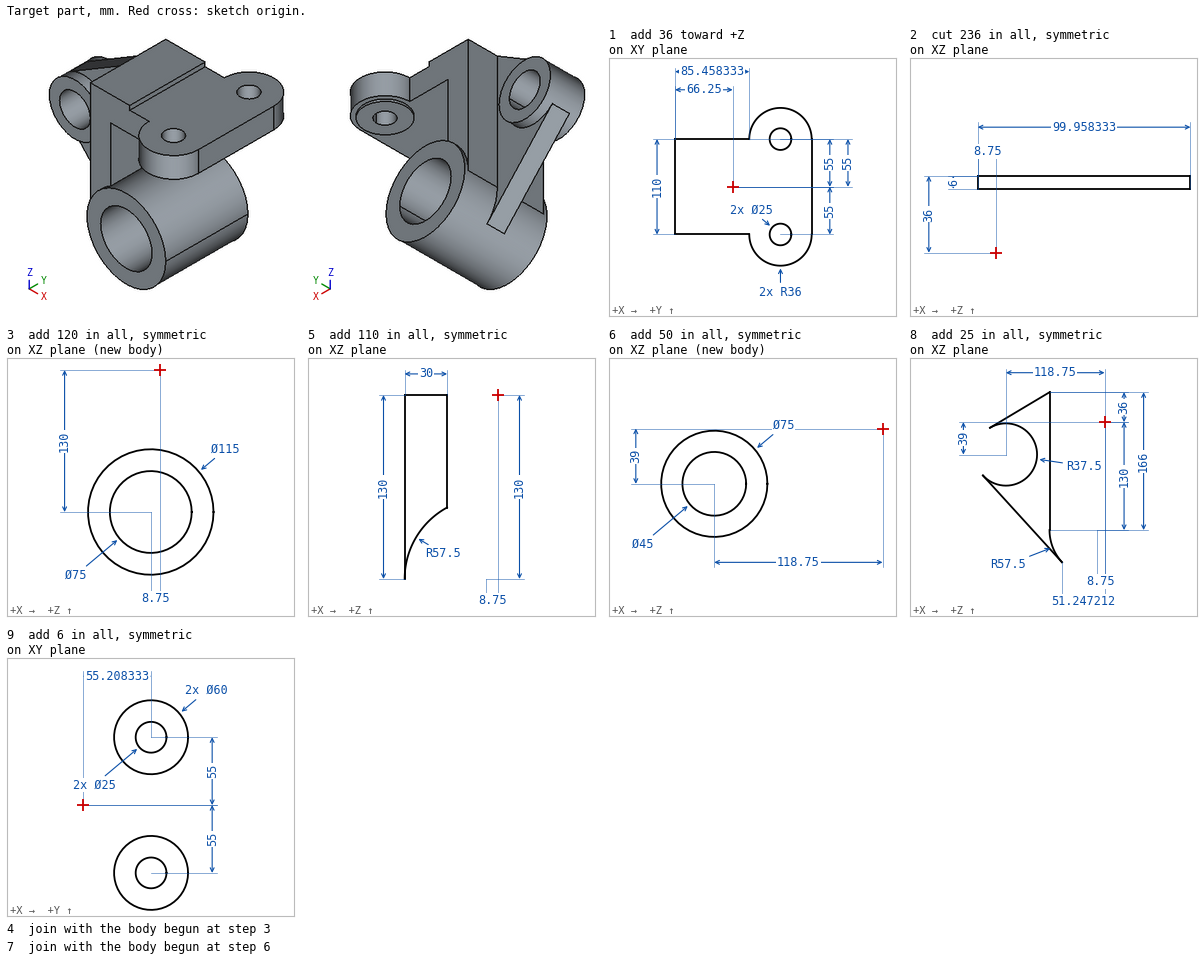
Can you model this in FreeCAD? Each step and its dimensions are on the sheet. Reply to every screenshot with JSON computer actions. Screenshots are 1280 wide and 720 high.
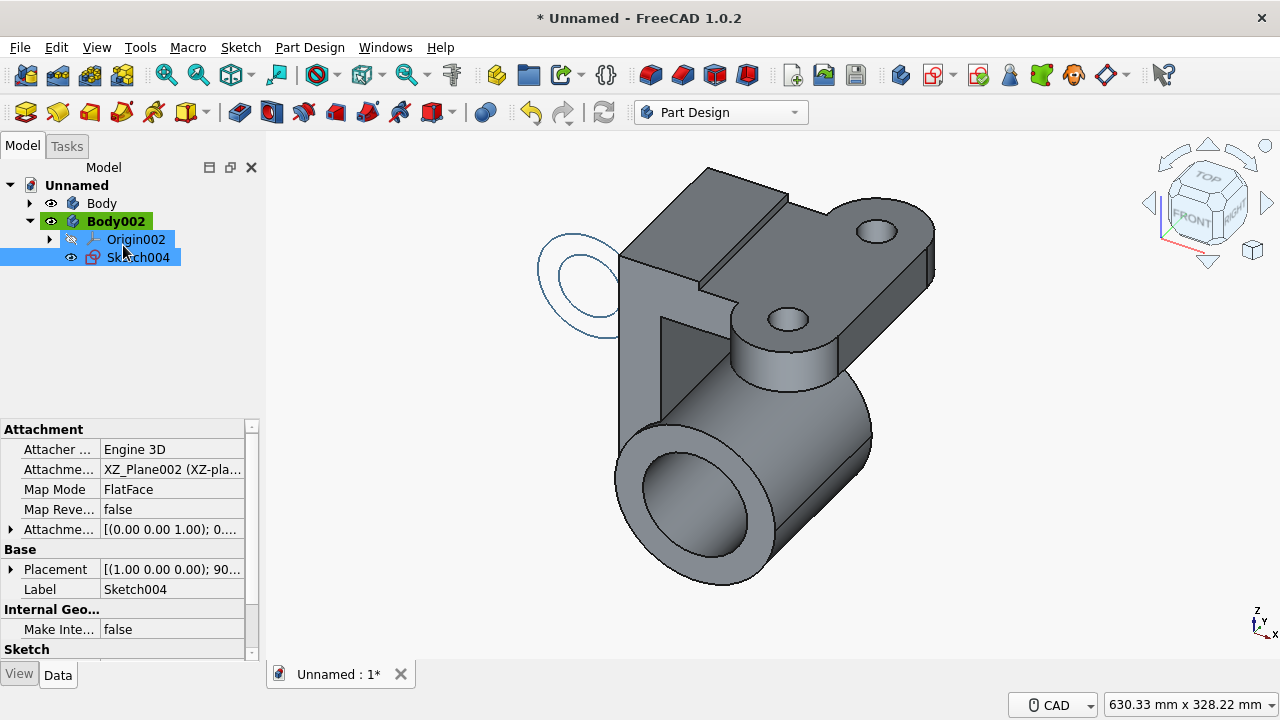
{"action": "left_click", "coordinate": [26, 112]}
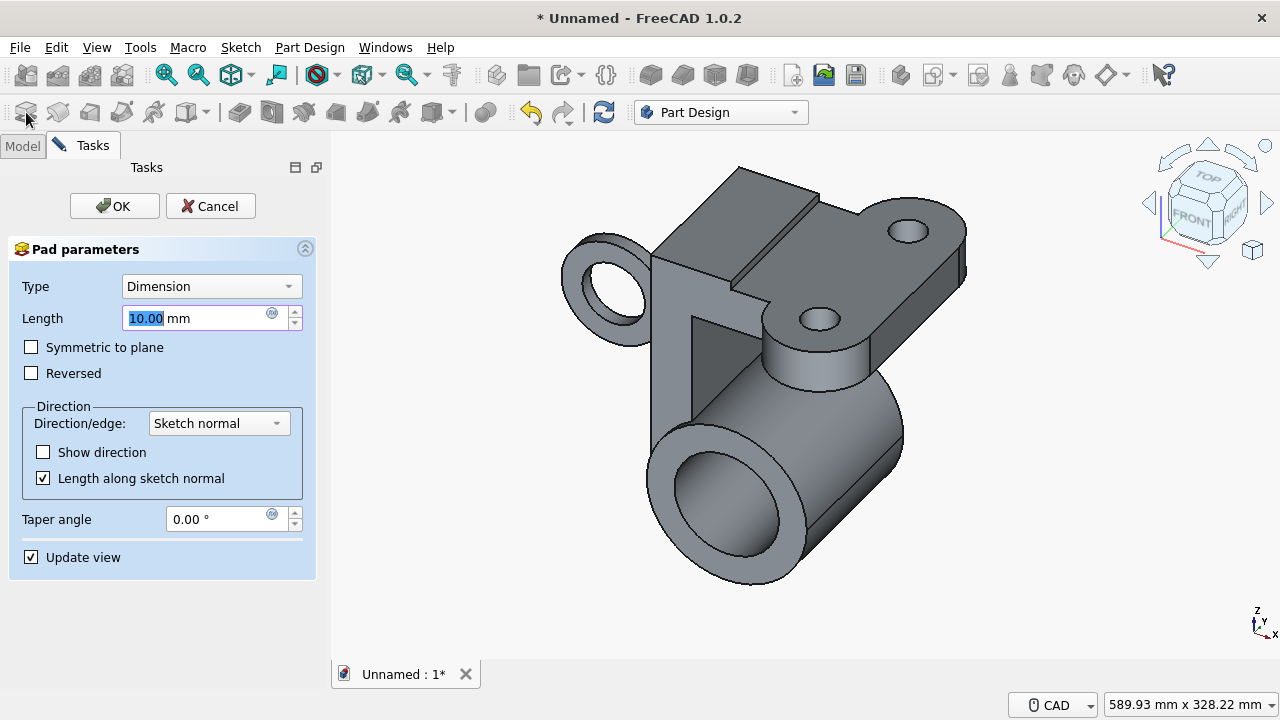
{"action": "type", "text": "50"}
{"action": "key", "text": "Tab"}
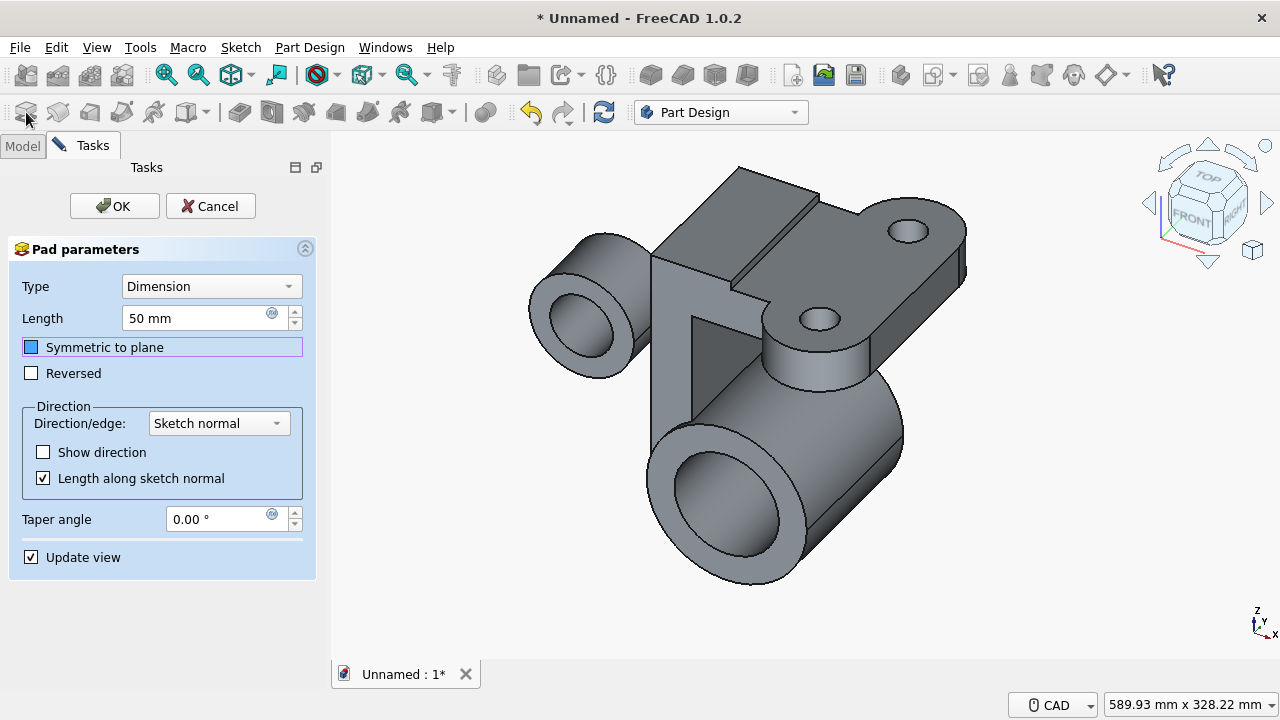
{"action": "left_click", "coordinate": [30, 347]}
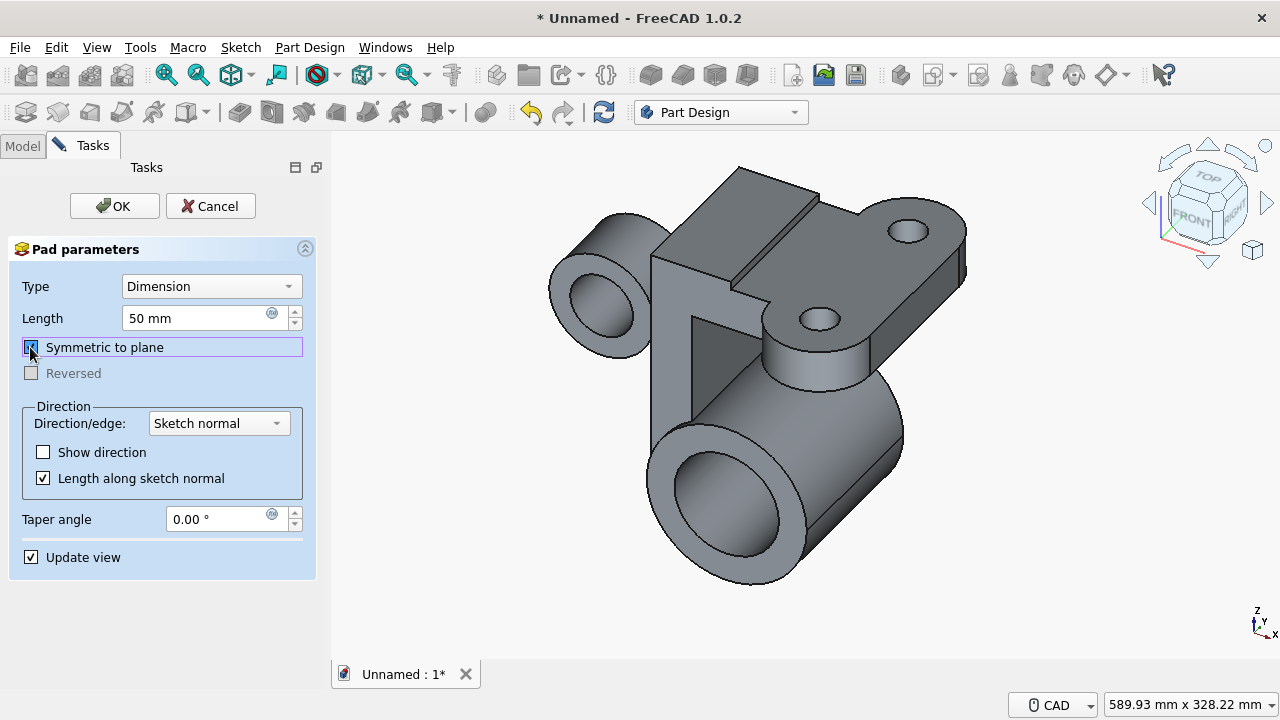
{"action": "left_click", "coordinate": [115, 206]}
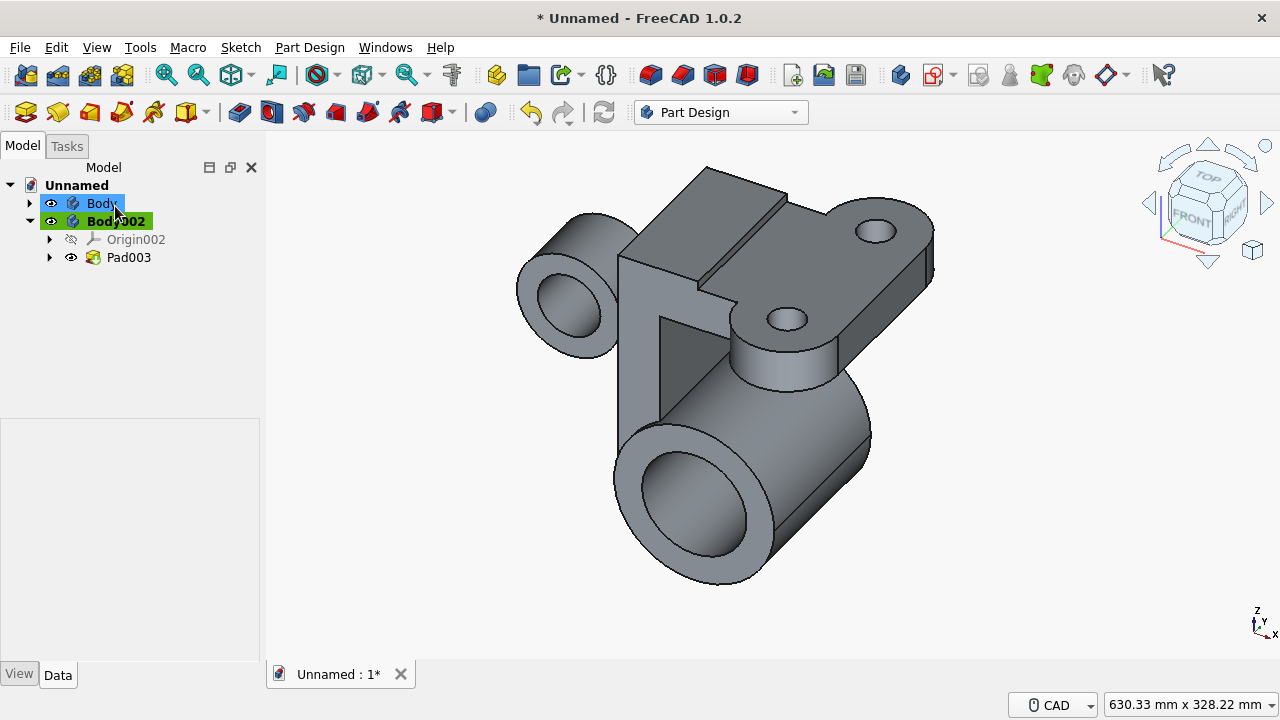
{"action": "key", "text": "v f"}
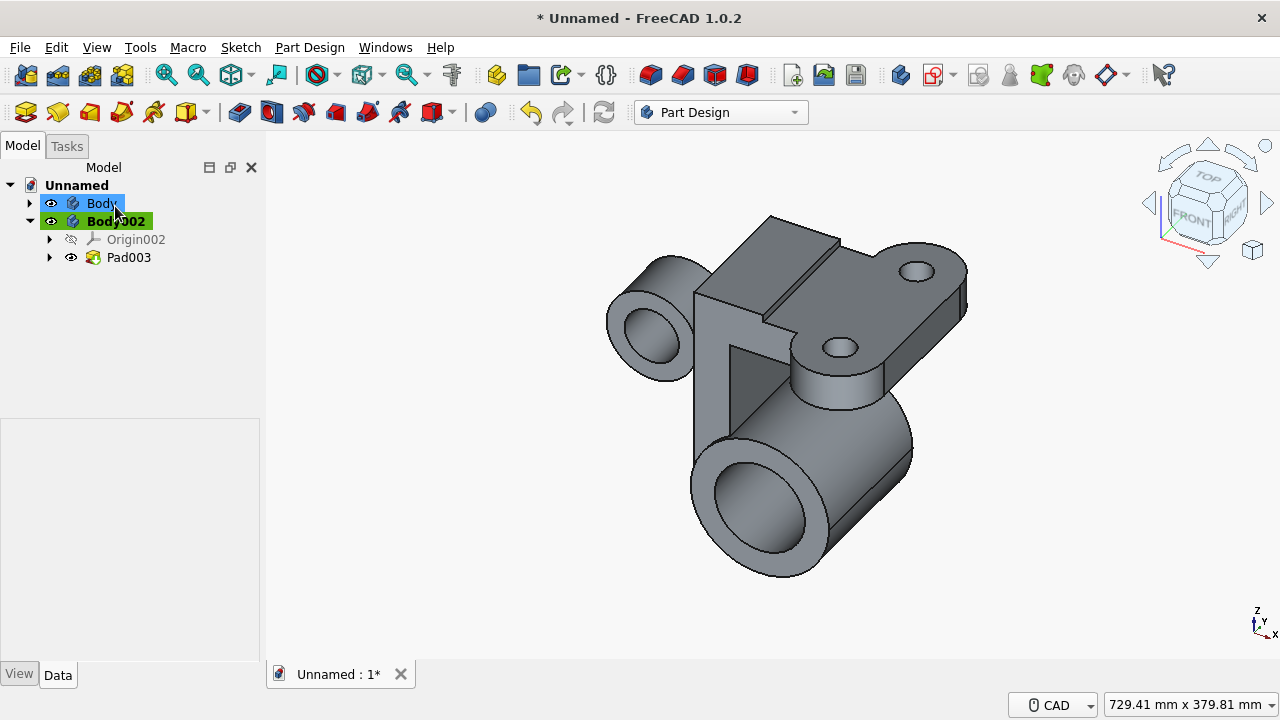
{"action": "double_click", "coordinate": [96, 203]}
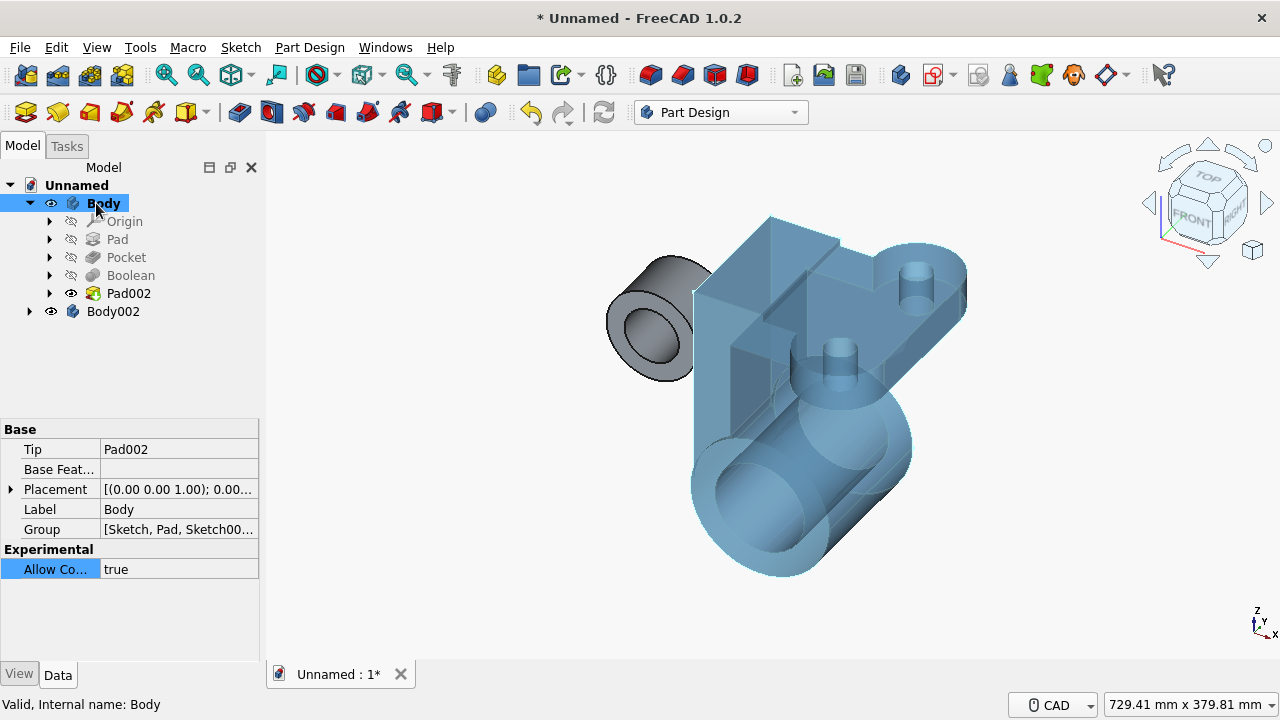
{"action": "left_click", "coordinate": [96, 311]}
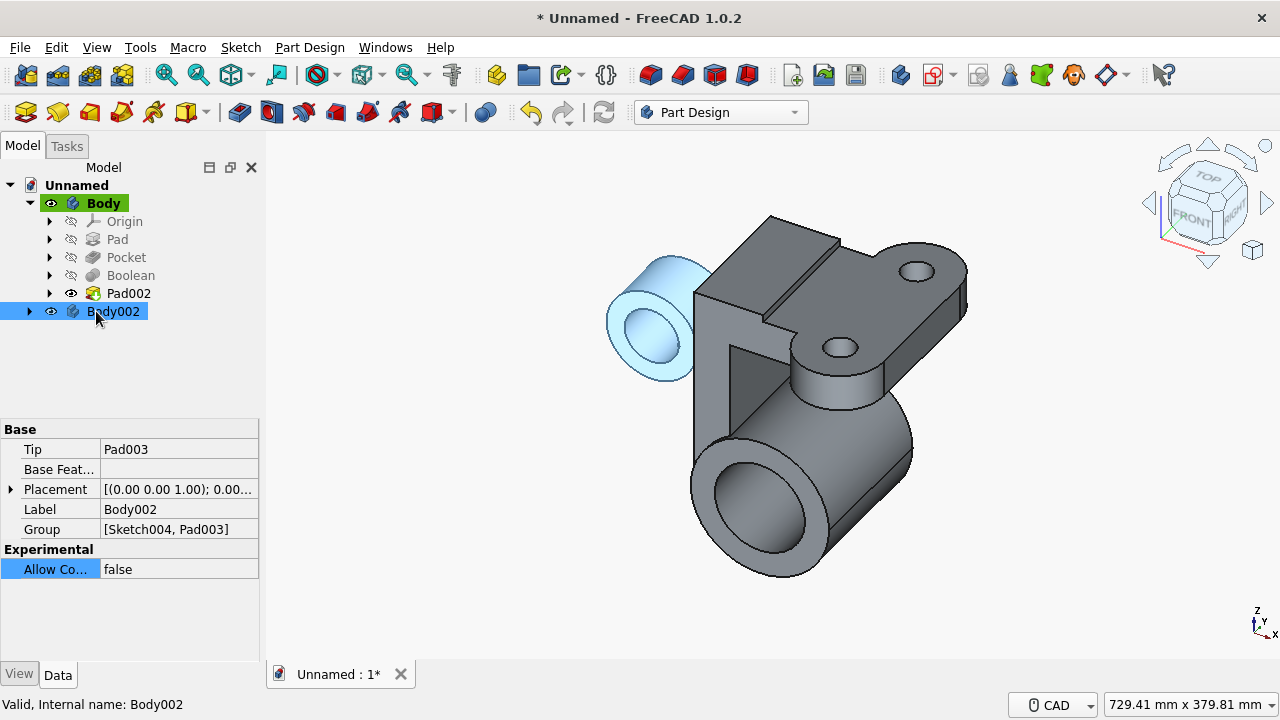
{"action": "left_click", "coordinate": [486, 112]}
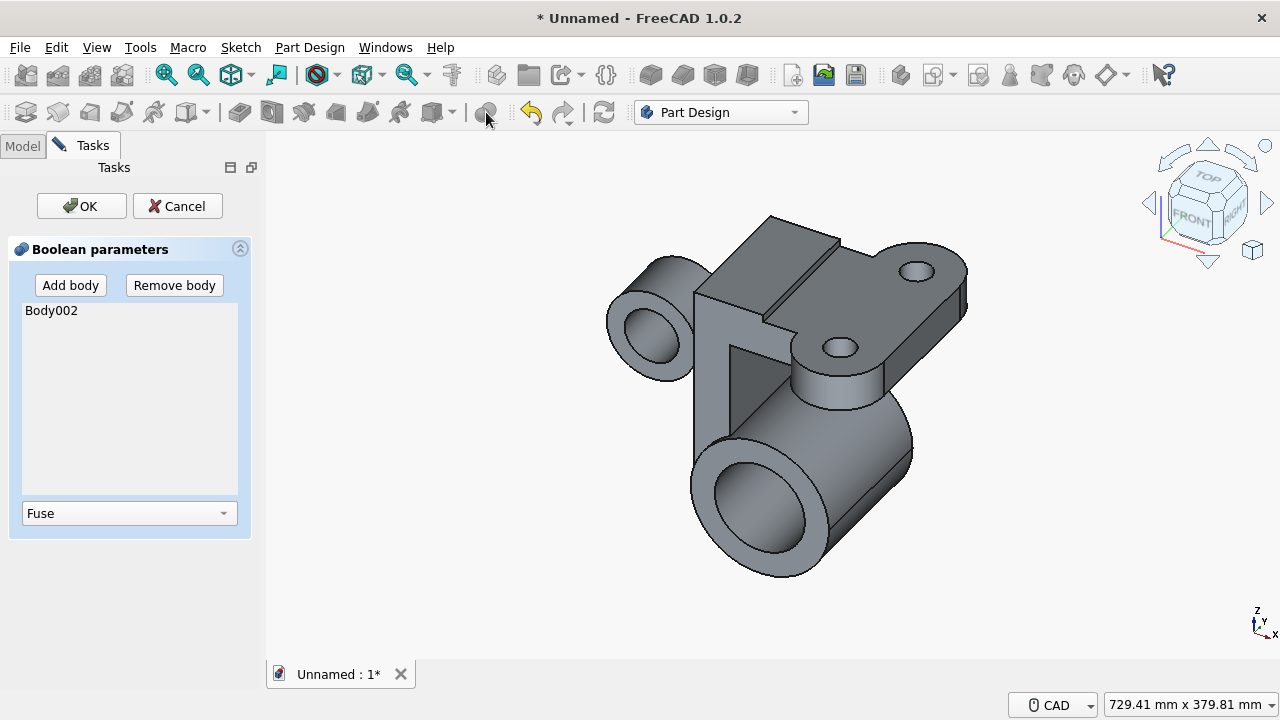
{"action": "left_click", "coordinate": [82, 206]}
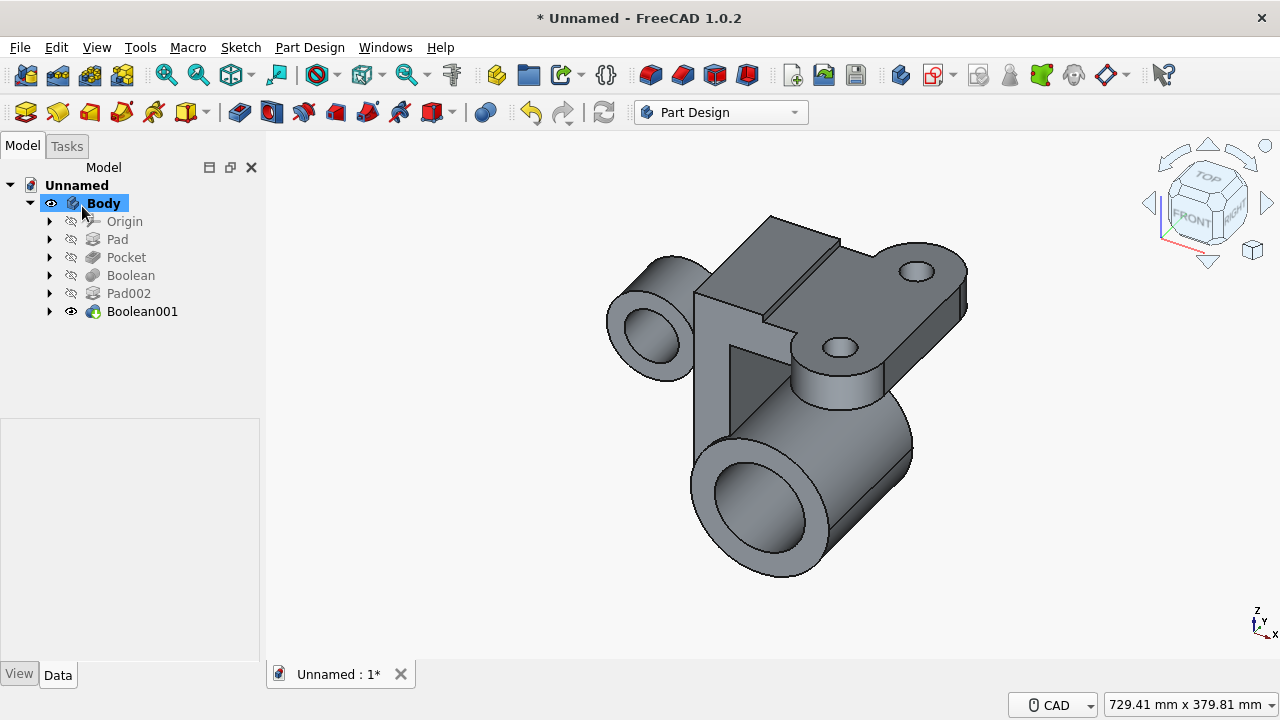
{"action": "left_click", "coordinate": [934, 76]}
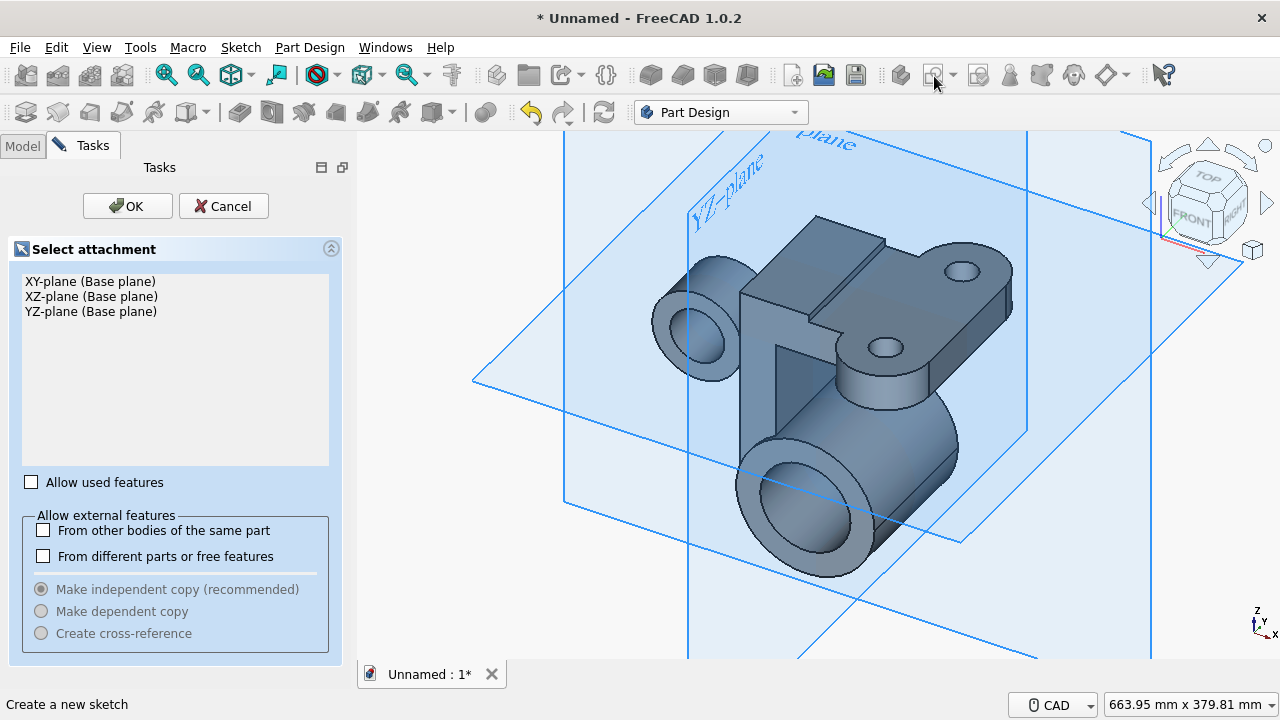
{"action": "left_click", "coordinate": [82, 296]}